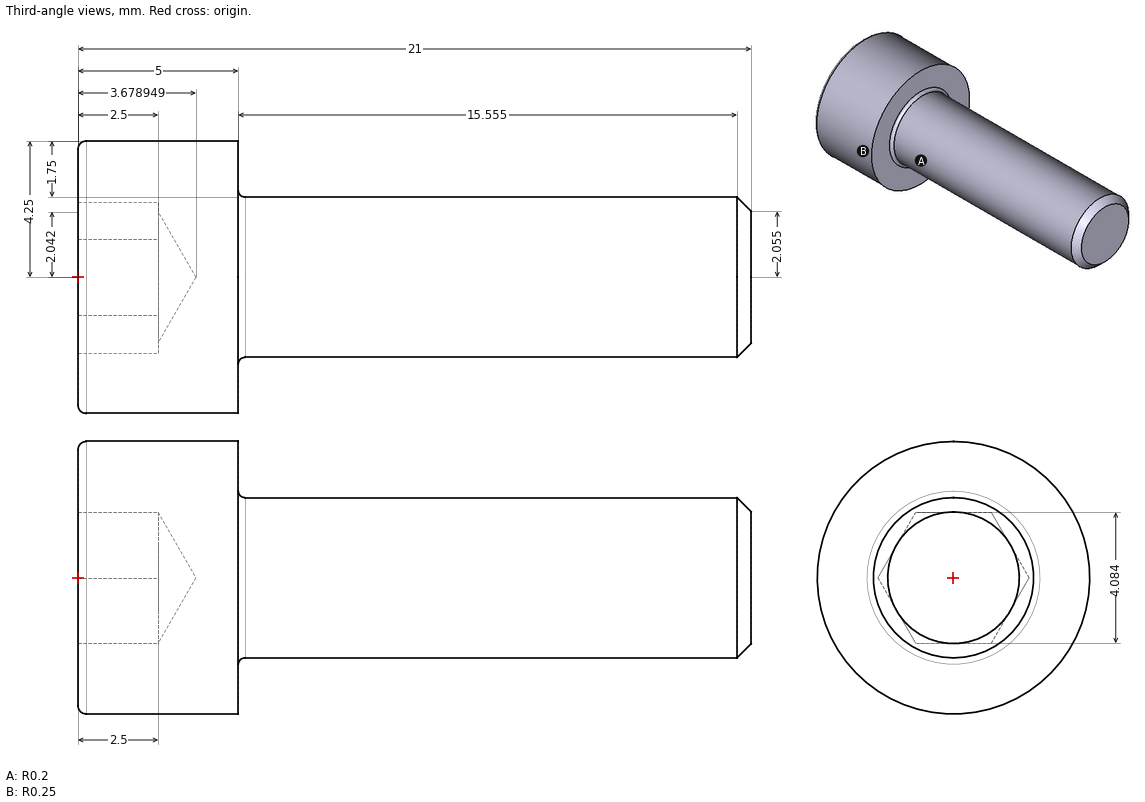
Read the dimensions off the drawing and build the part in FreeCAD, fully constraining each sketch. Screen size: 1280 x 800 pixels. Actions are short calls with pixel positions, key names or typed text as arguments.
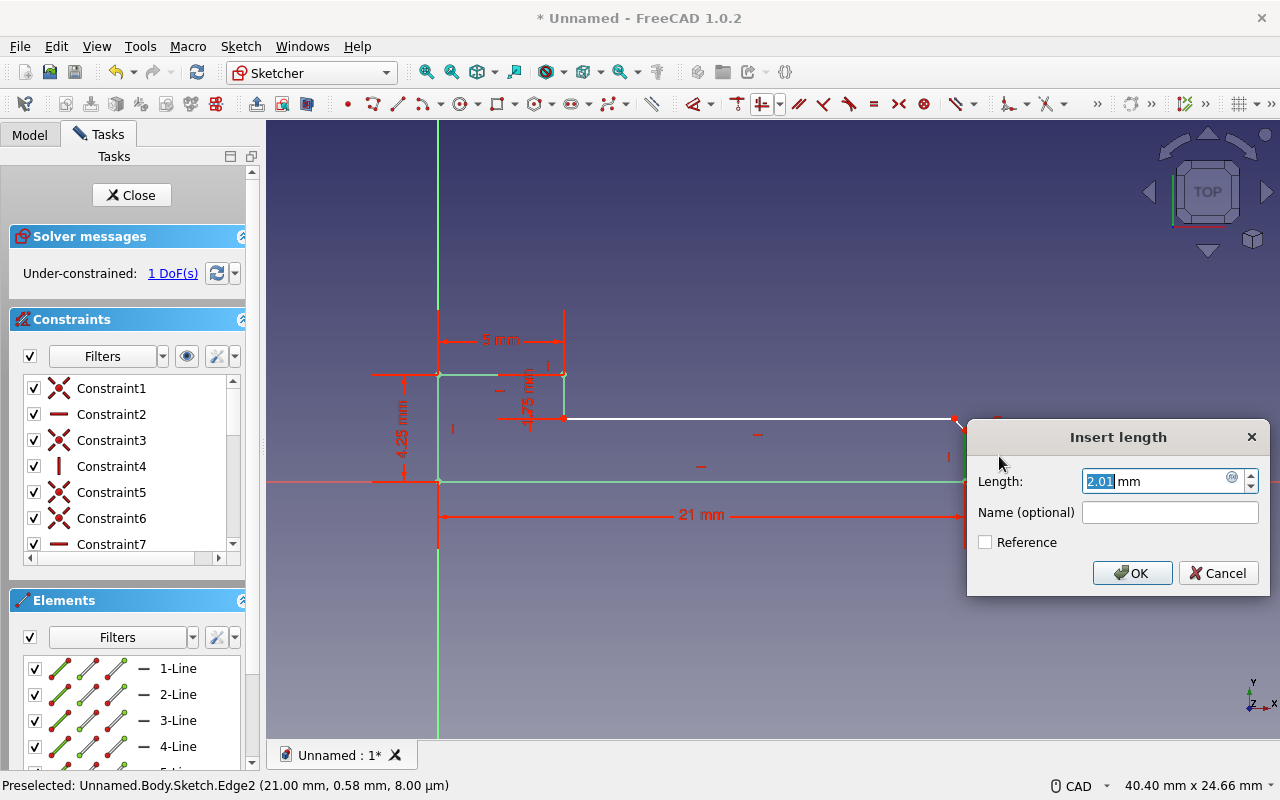
text(2.055)
key(Return)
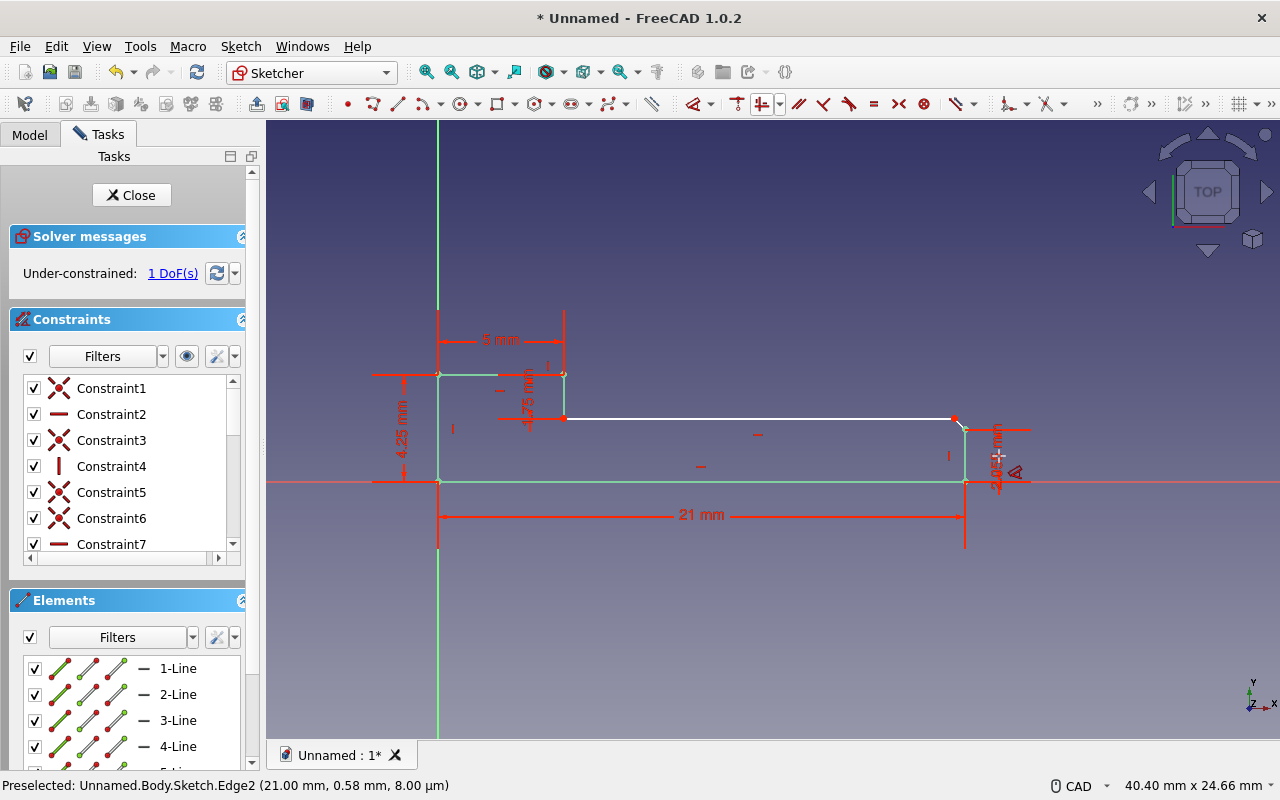
click(837, 419)
click(759, 385)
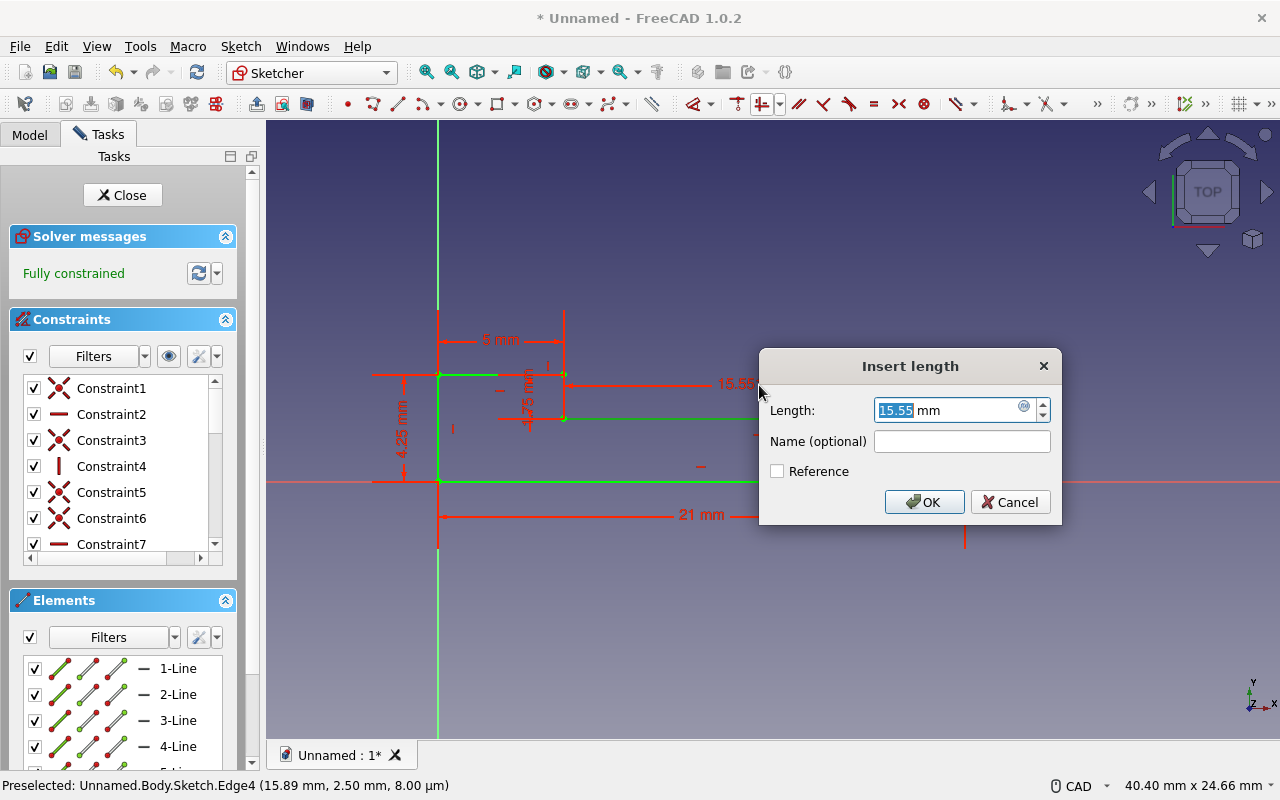
text(15.555)
key(Return)
key(Escape)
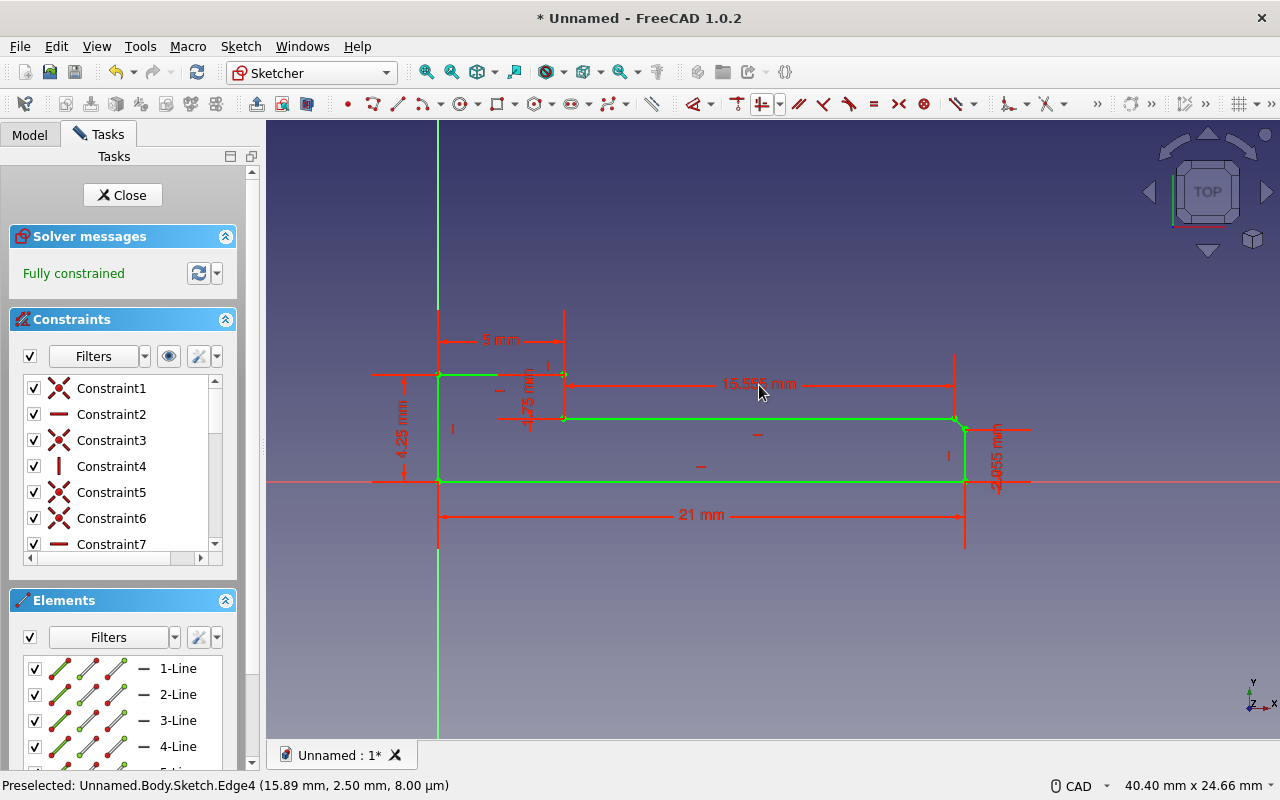
click(123, 195)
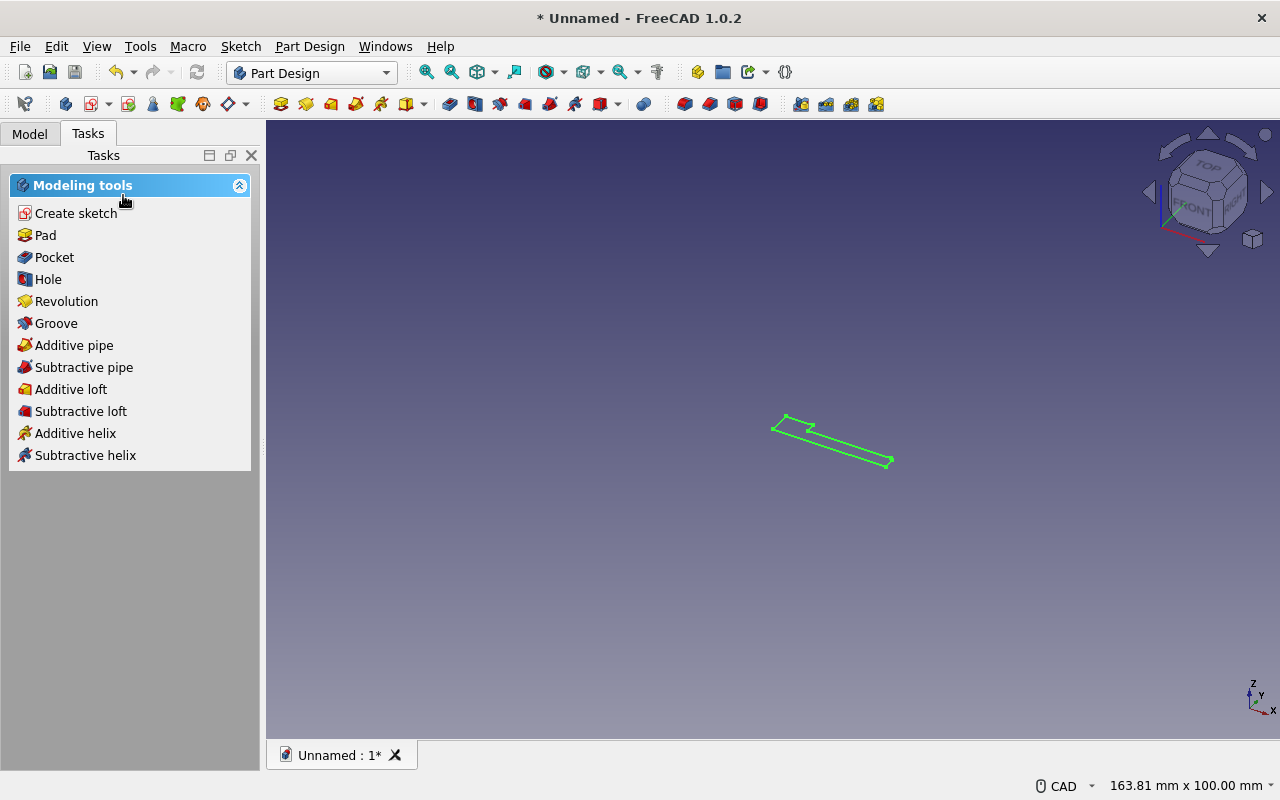
click(306, 104)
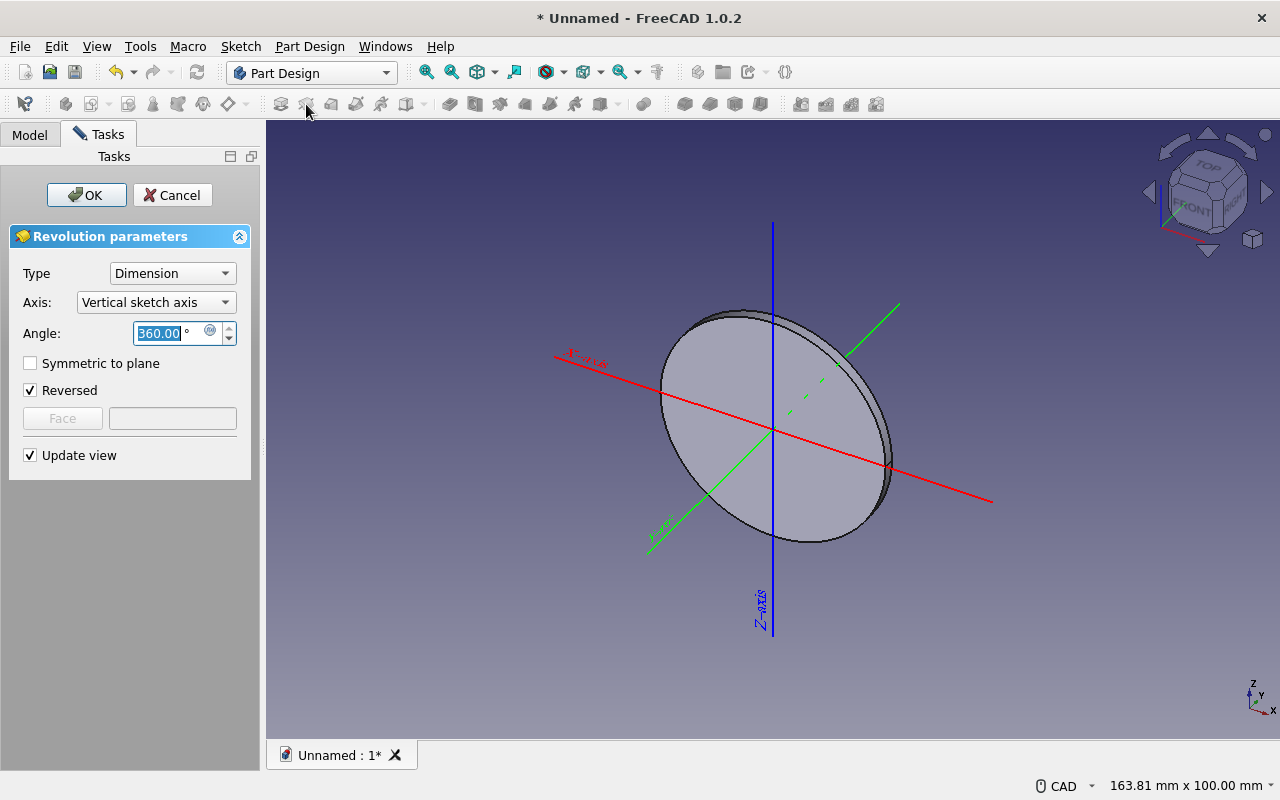
click(157, 302)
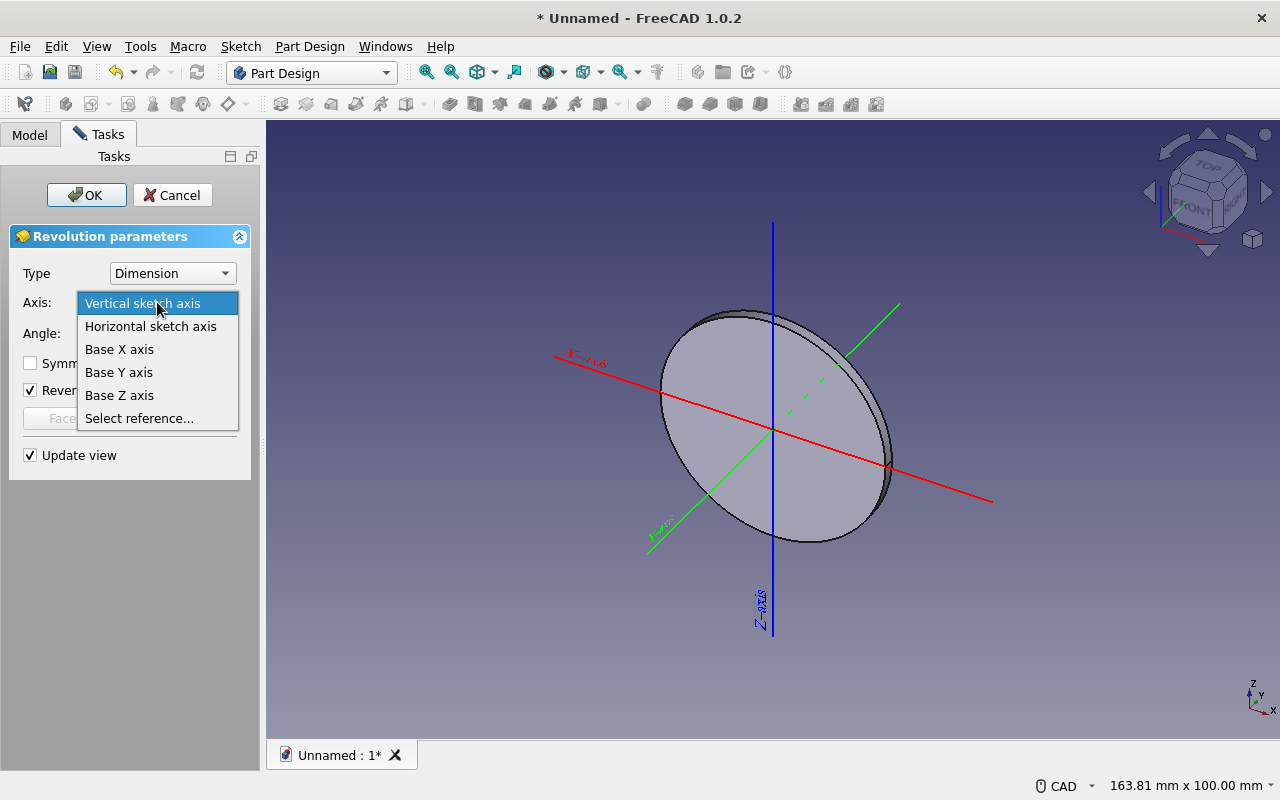
click(156, 326)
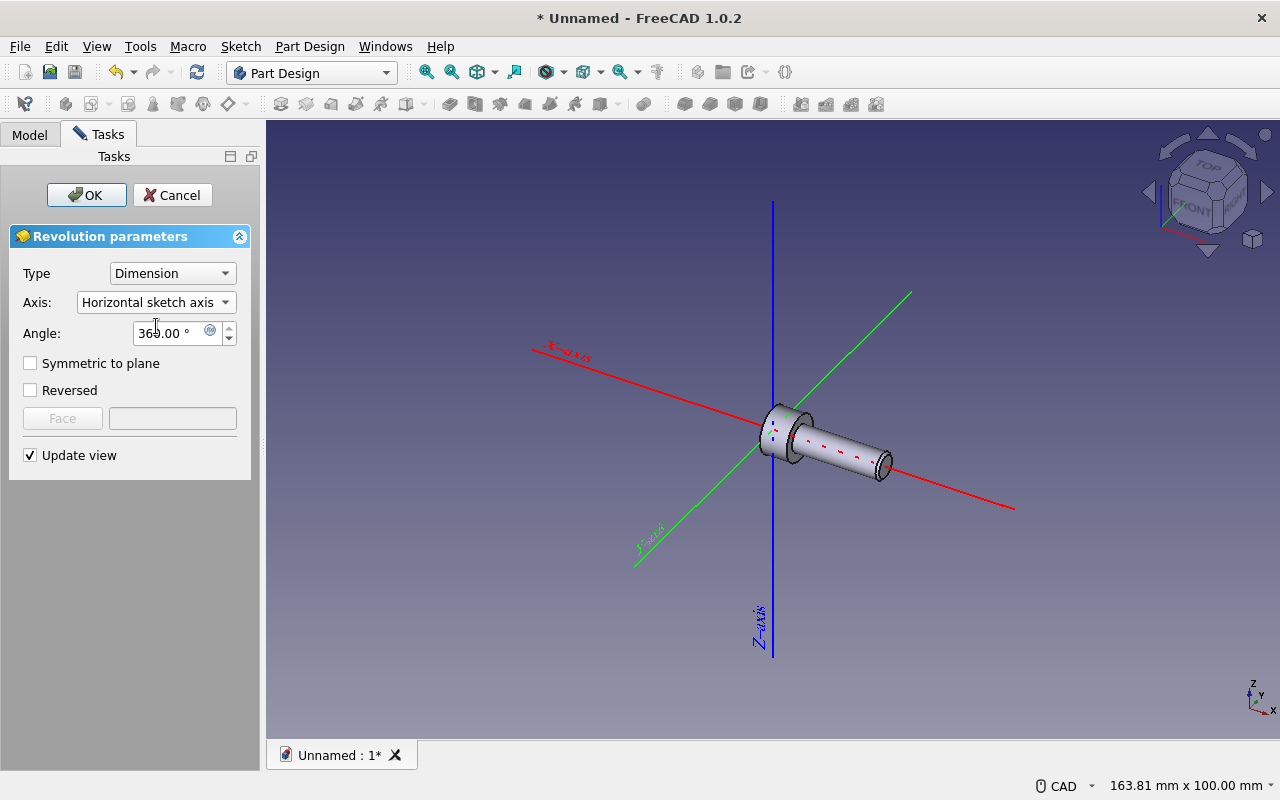
click(87, 195)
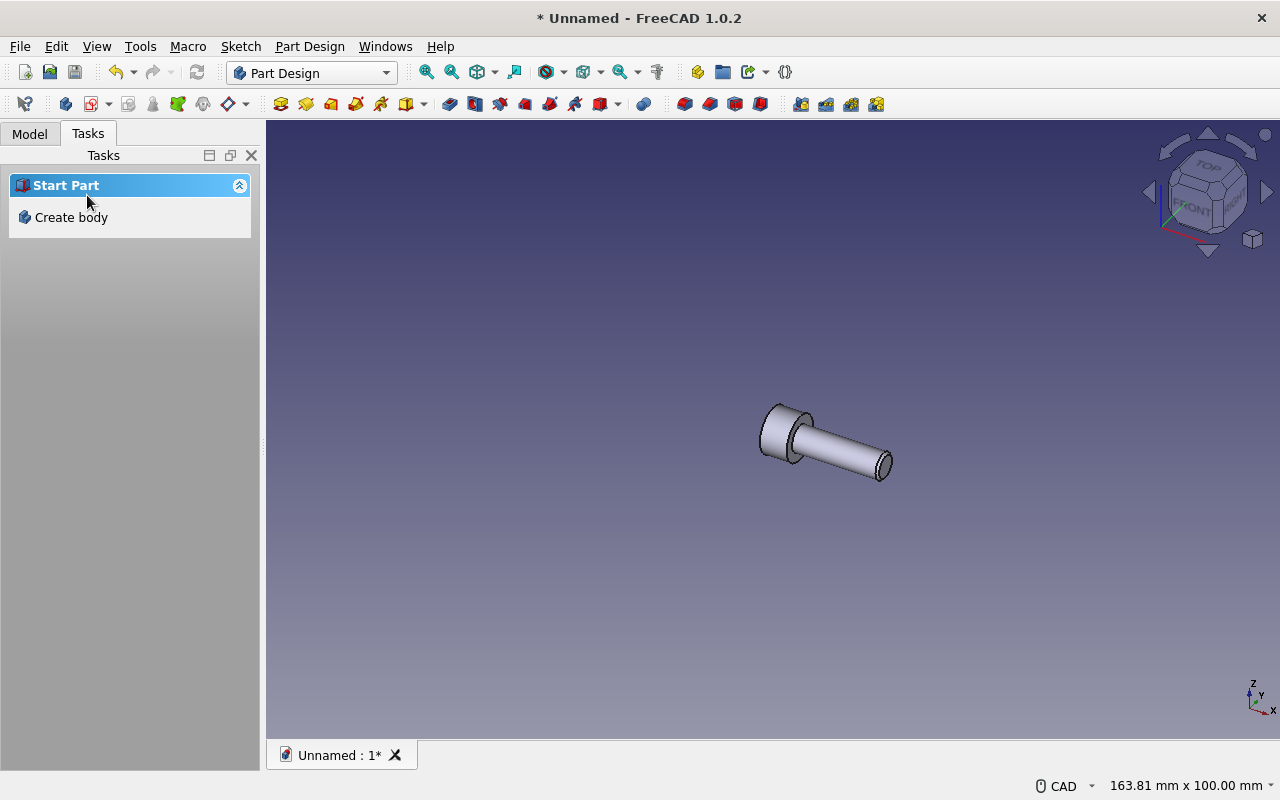
click(427, 72)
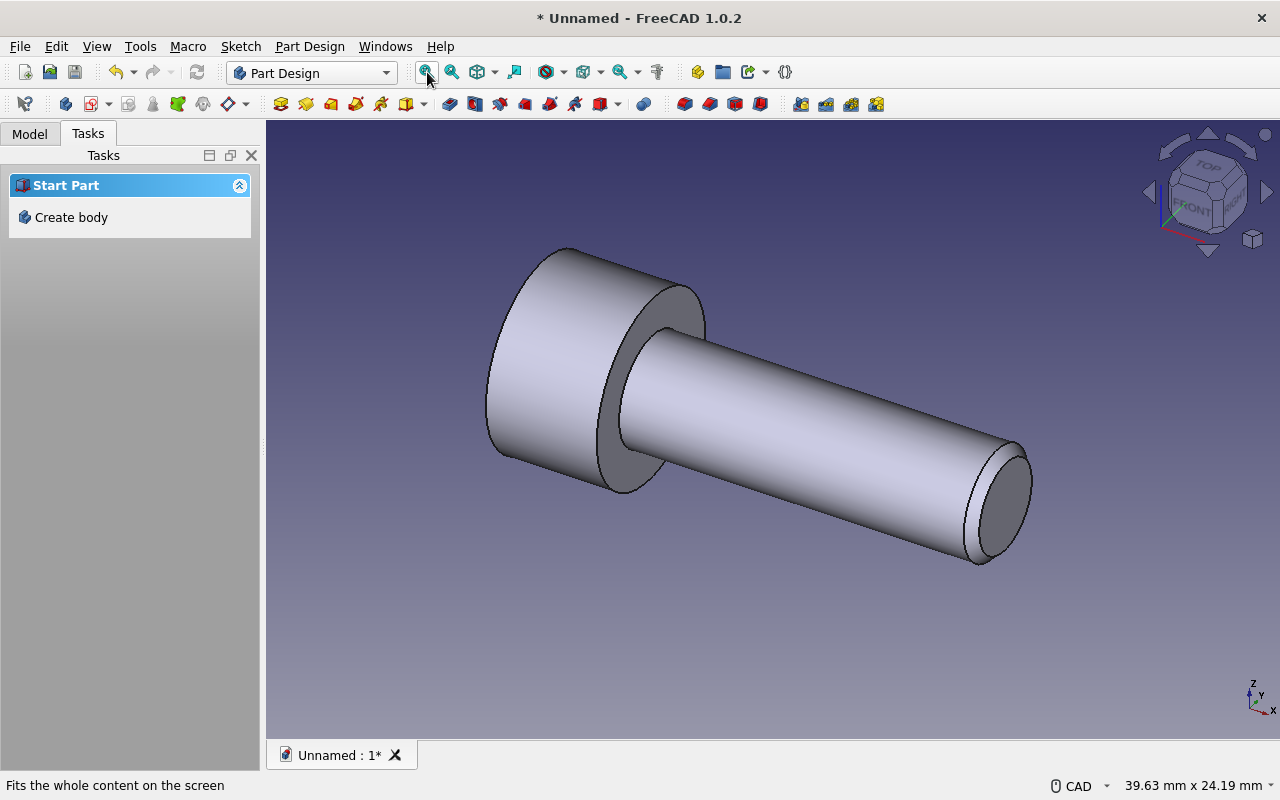
key(0)